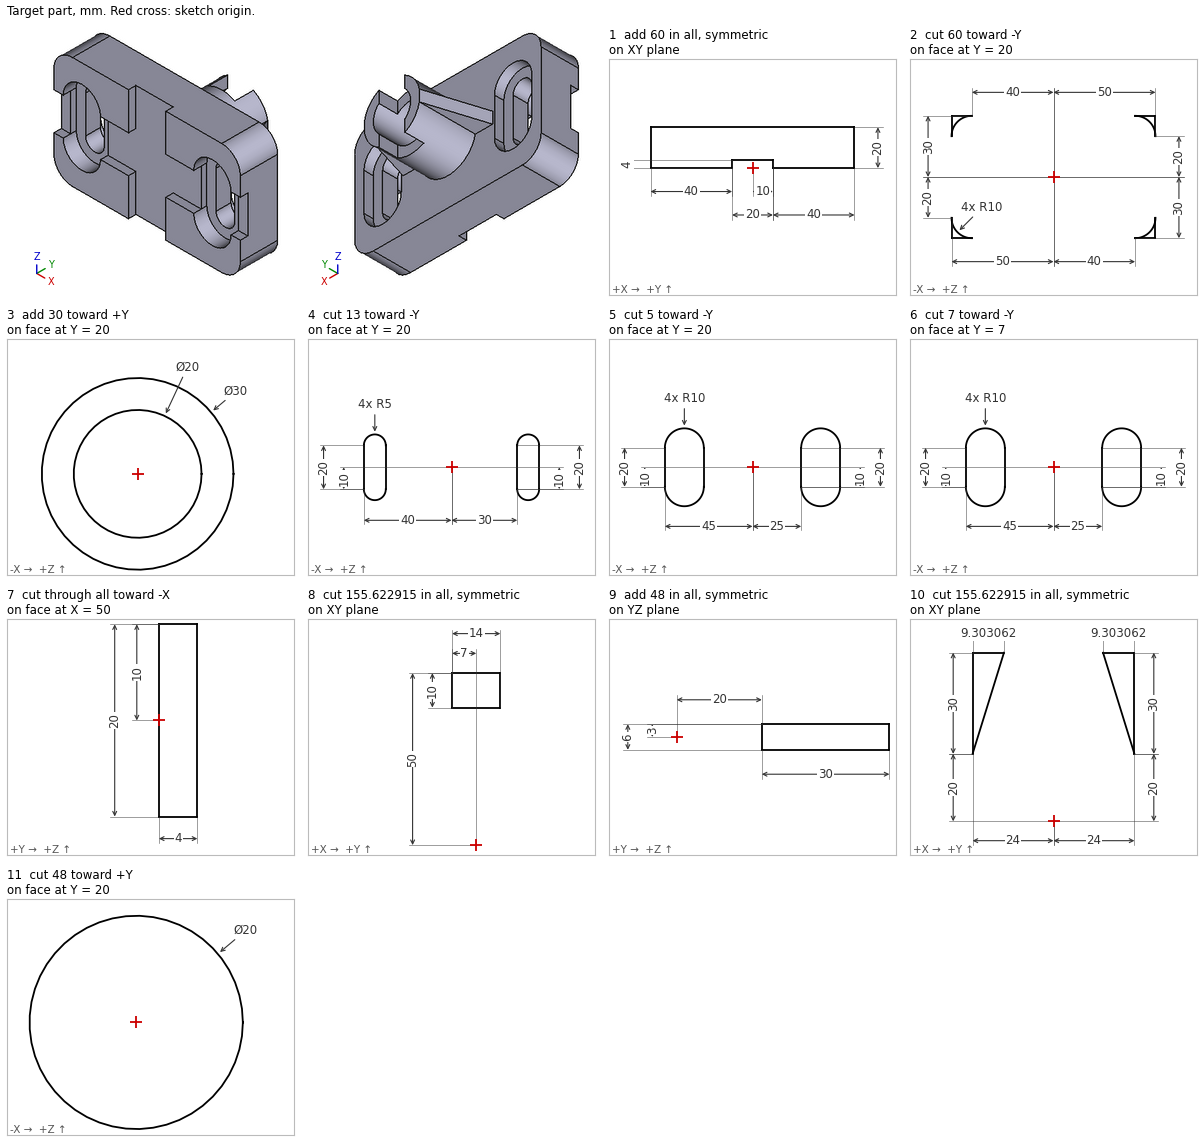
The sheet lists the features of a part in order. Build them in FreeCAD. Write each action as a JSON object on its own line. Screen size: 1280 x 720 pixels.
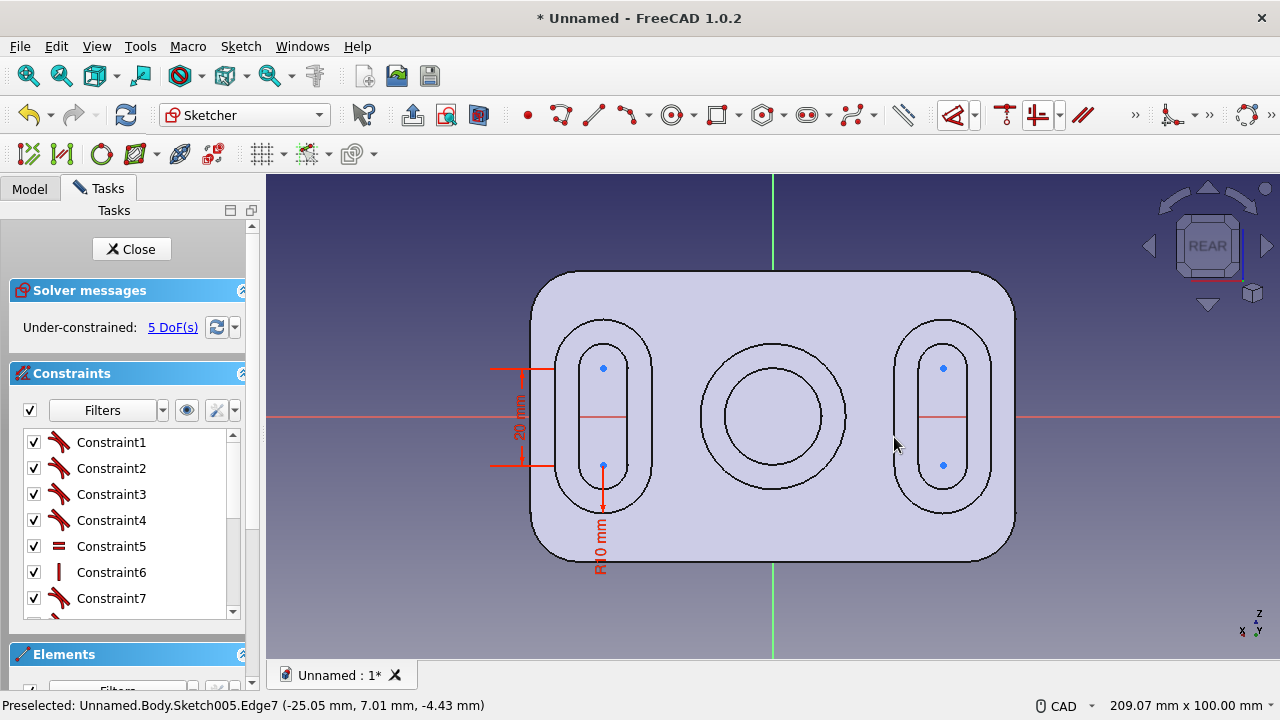
{"action": "key", "text": "i"}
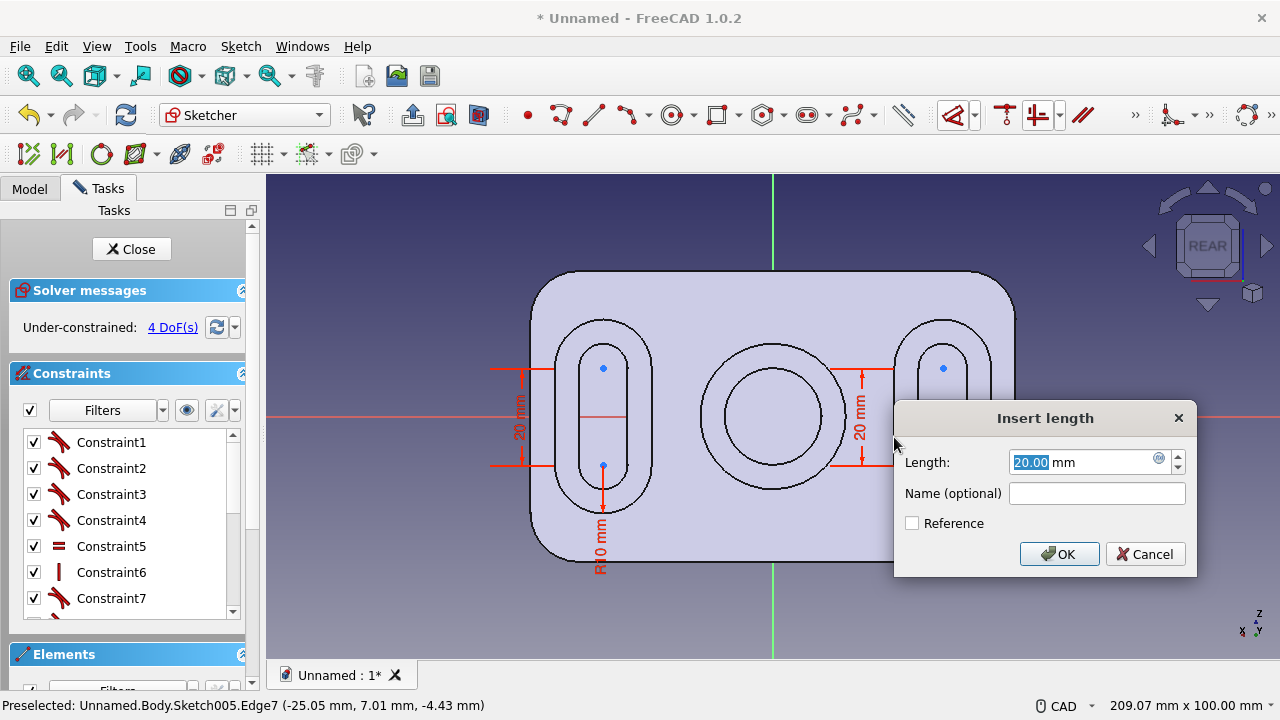
{"action": "type", "text": "20"}
{"action": "key", "text": "Return"}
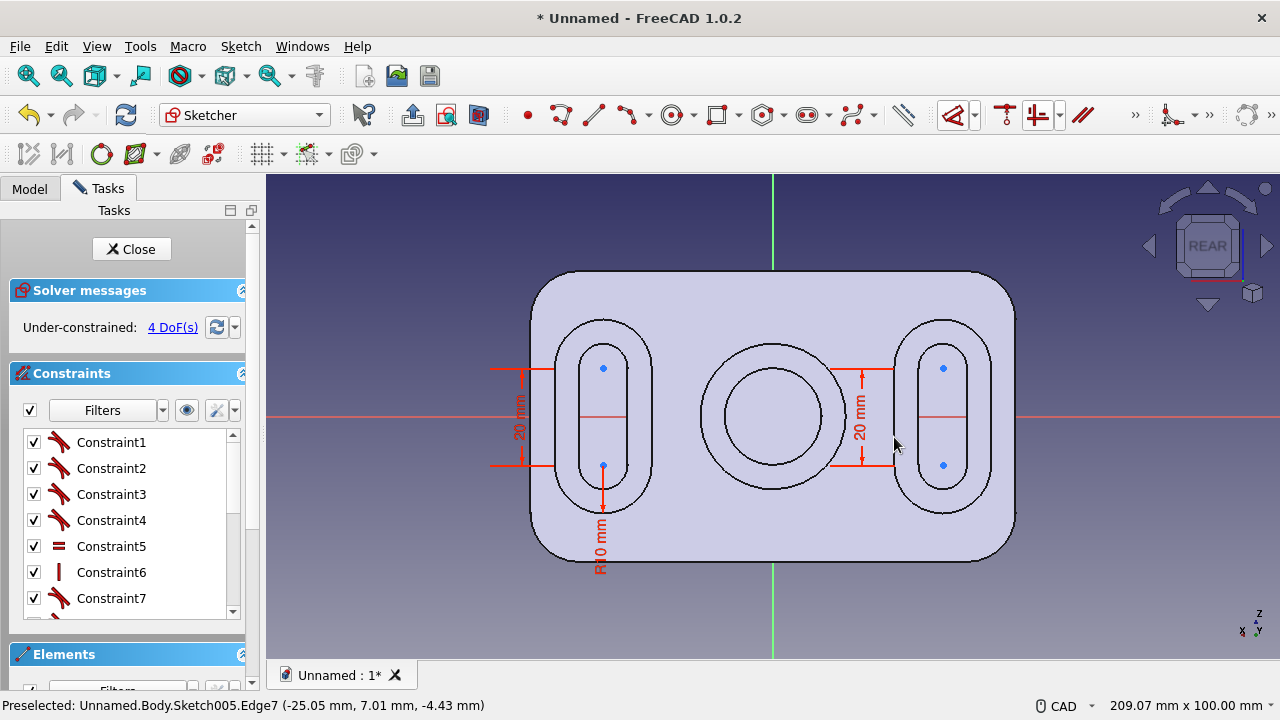
{"action": "left_click", "coordinate": [555, 466]}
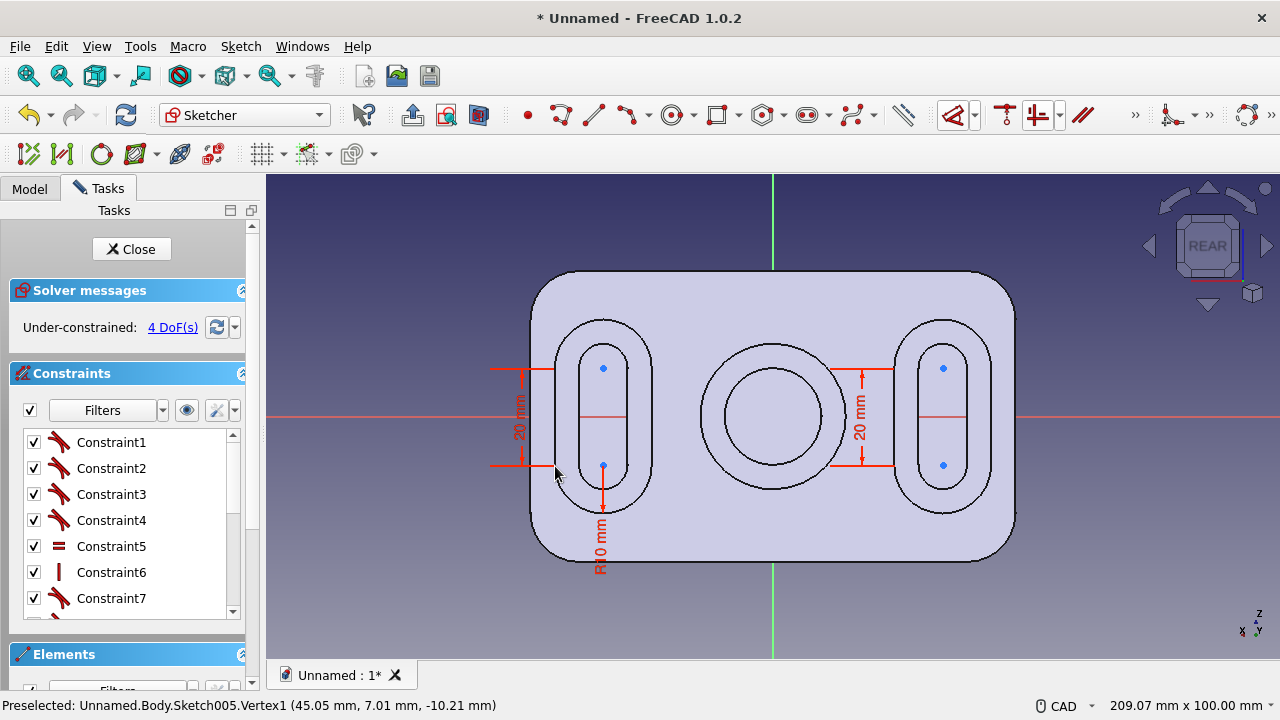
{"action": "key", "text": "l"}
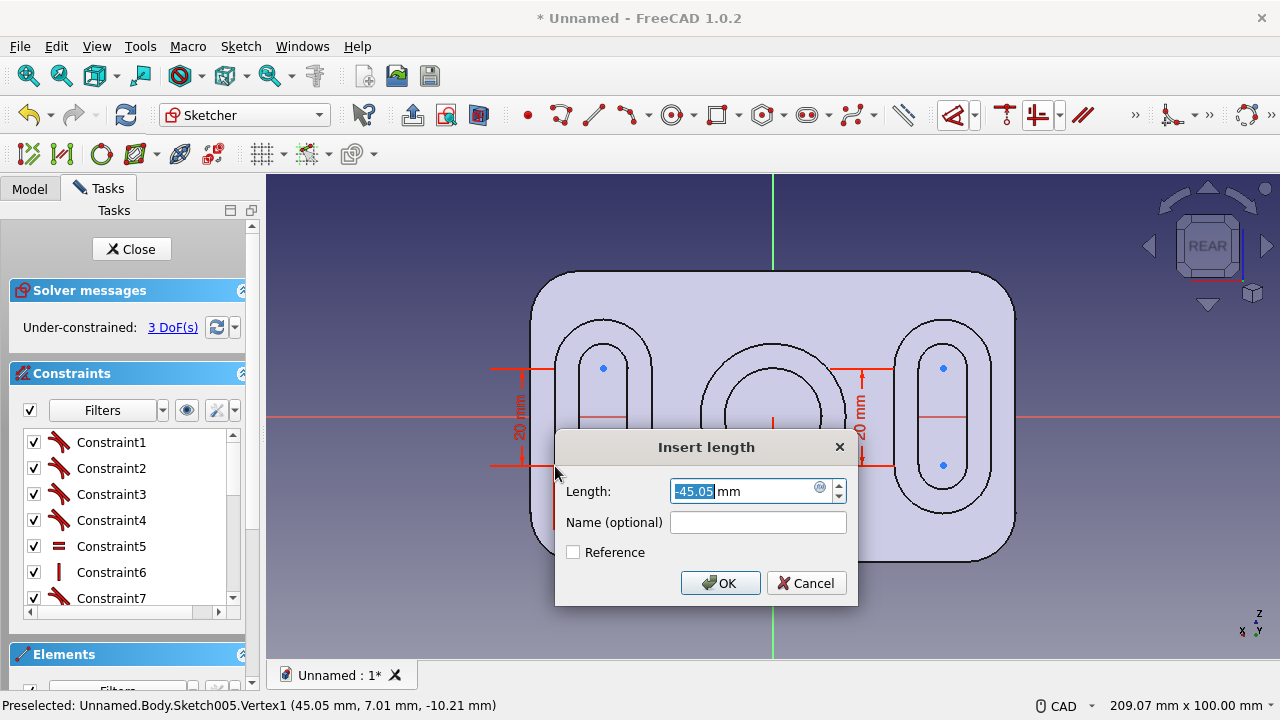
{"action": "type", "text": "-45"}
{"action": "key", "text": "Return"}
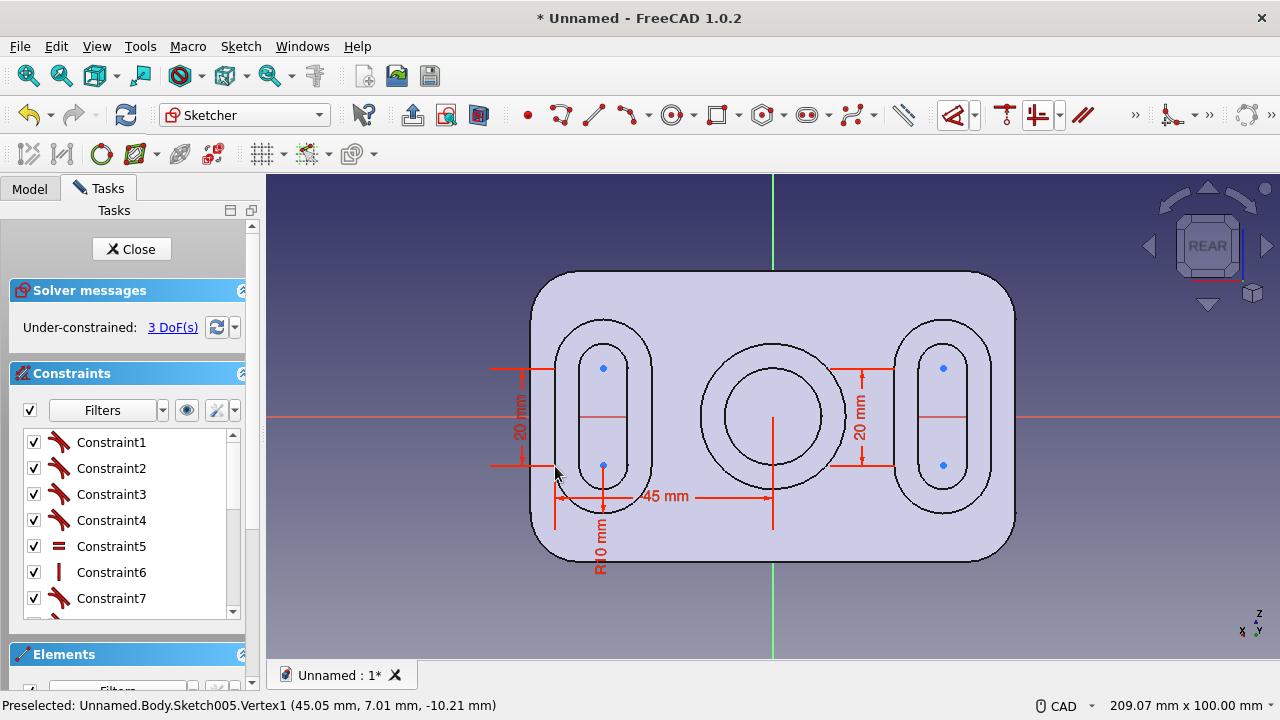
{"action": "left_click", "coordinate": [555, 466]}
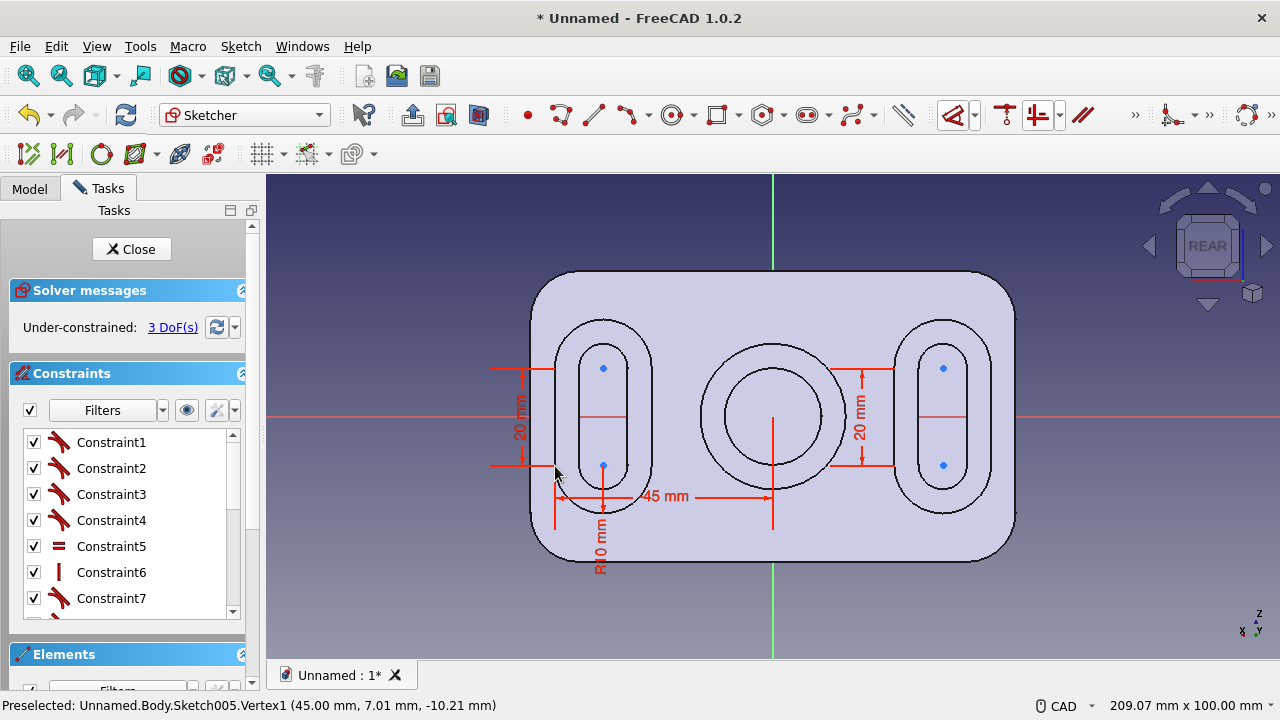
{"action": "key", "text": "i"}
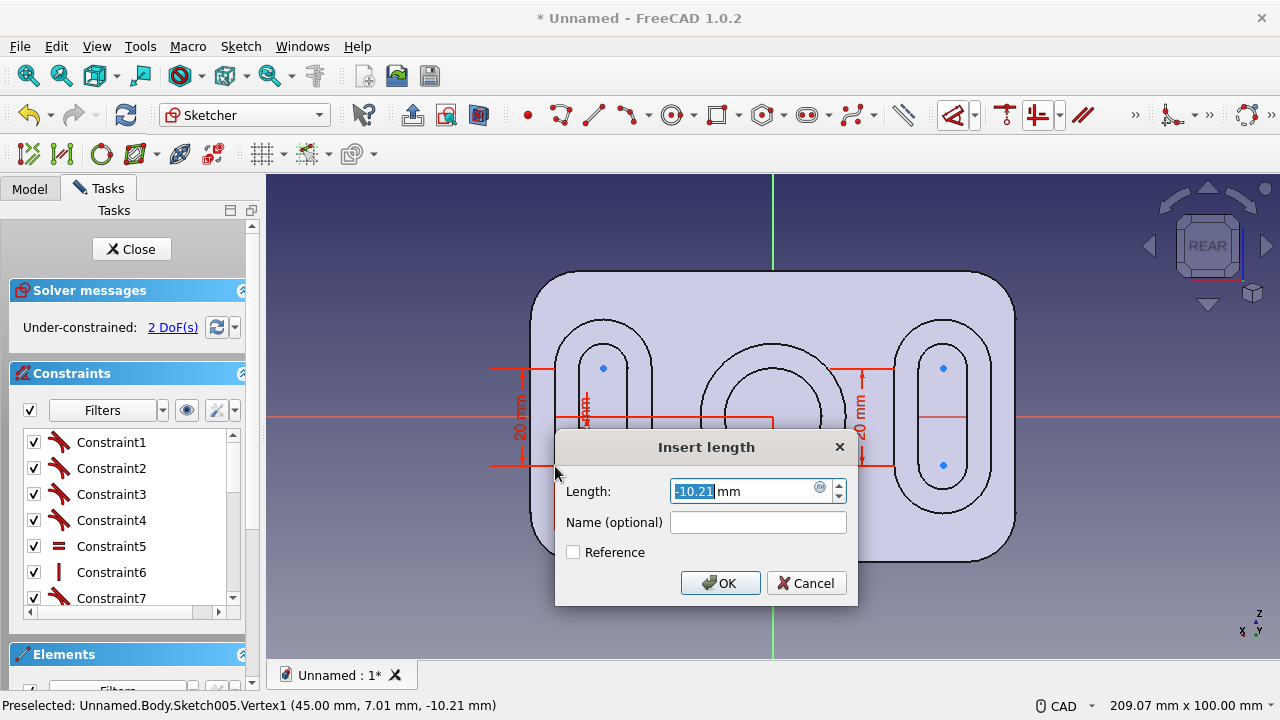
{"action": "type", "text": "-10"}
{"action": "key", "text": "Return"}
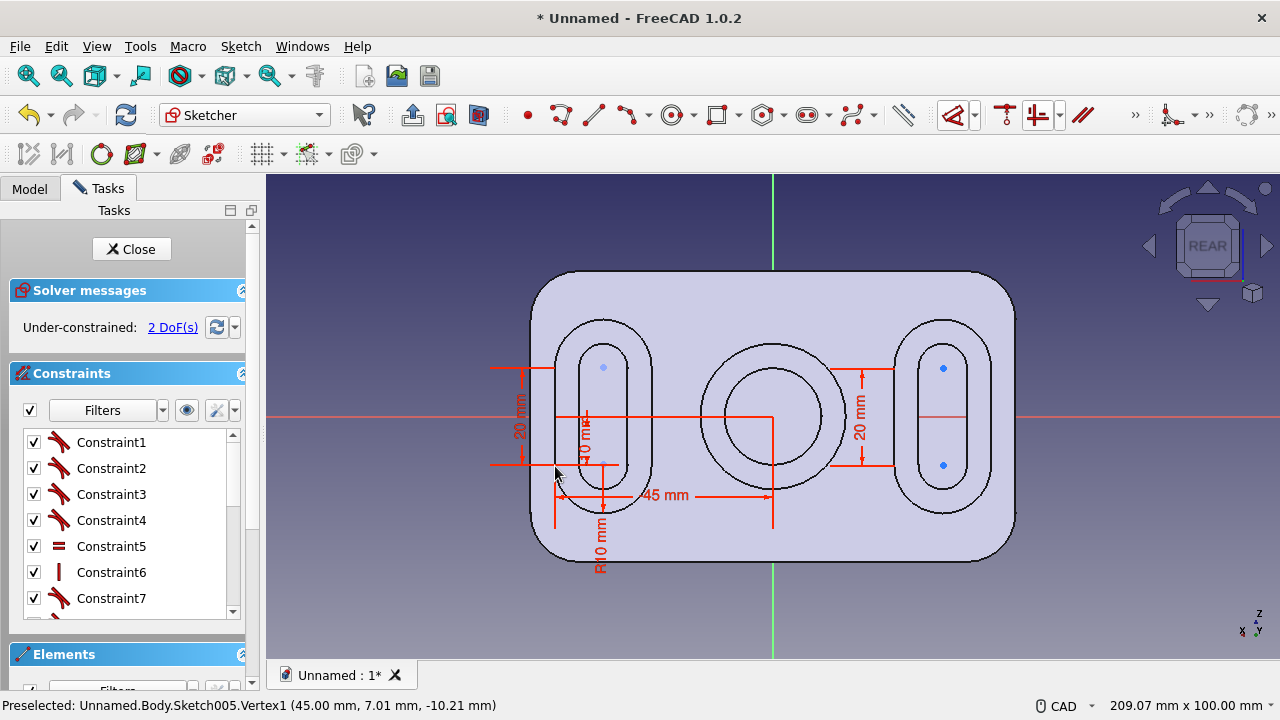
{"action": "left_click", "coordinate": [894, 466]}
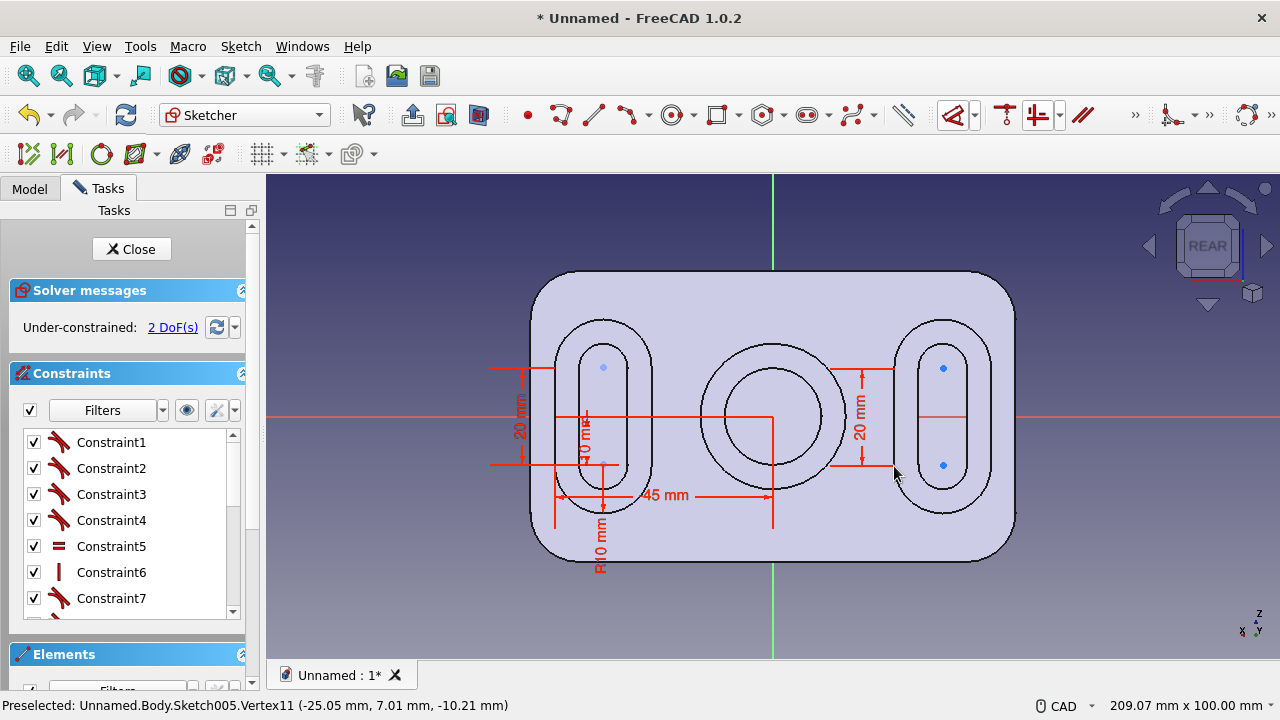
{"action": "key", "text": "l"}